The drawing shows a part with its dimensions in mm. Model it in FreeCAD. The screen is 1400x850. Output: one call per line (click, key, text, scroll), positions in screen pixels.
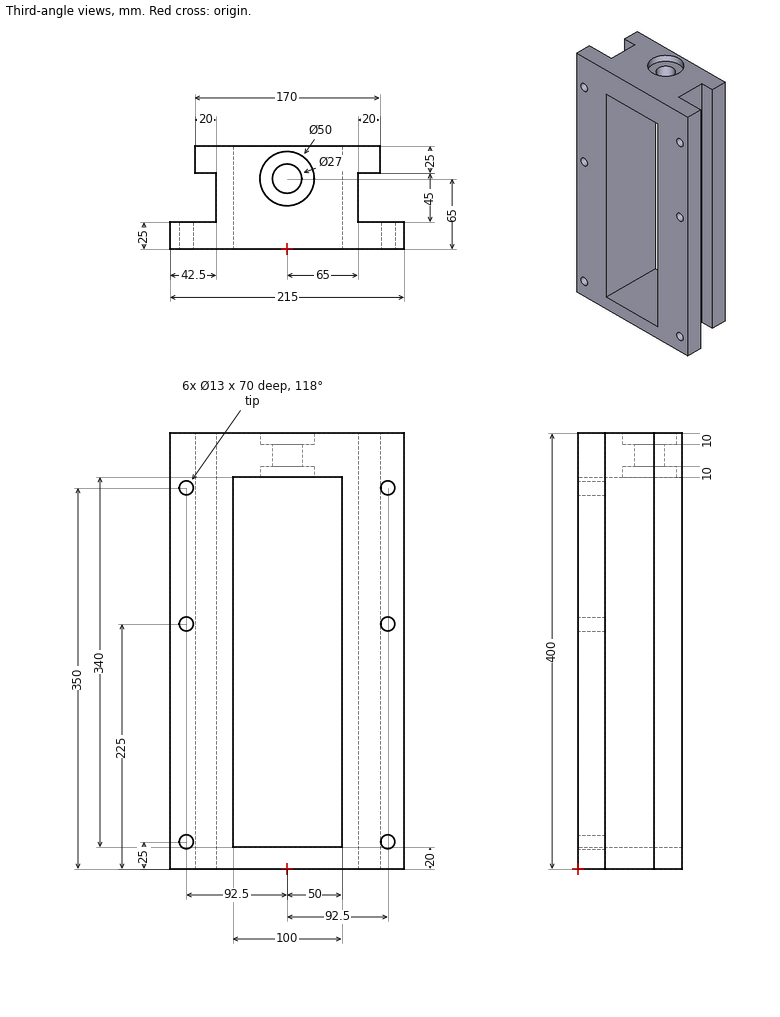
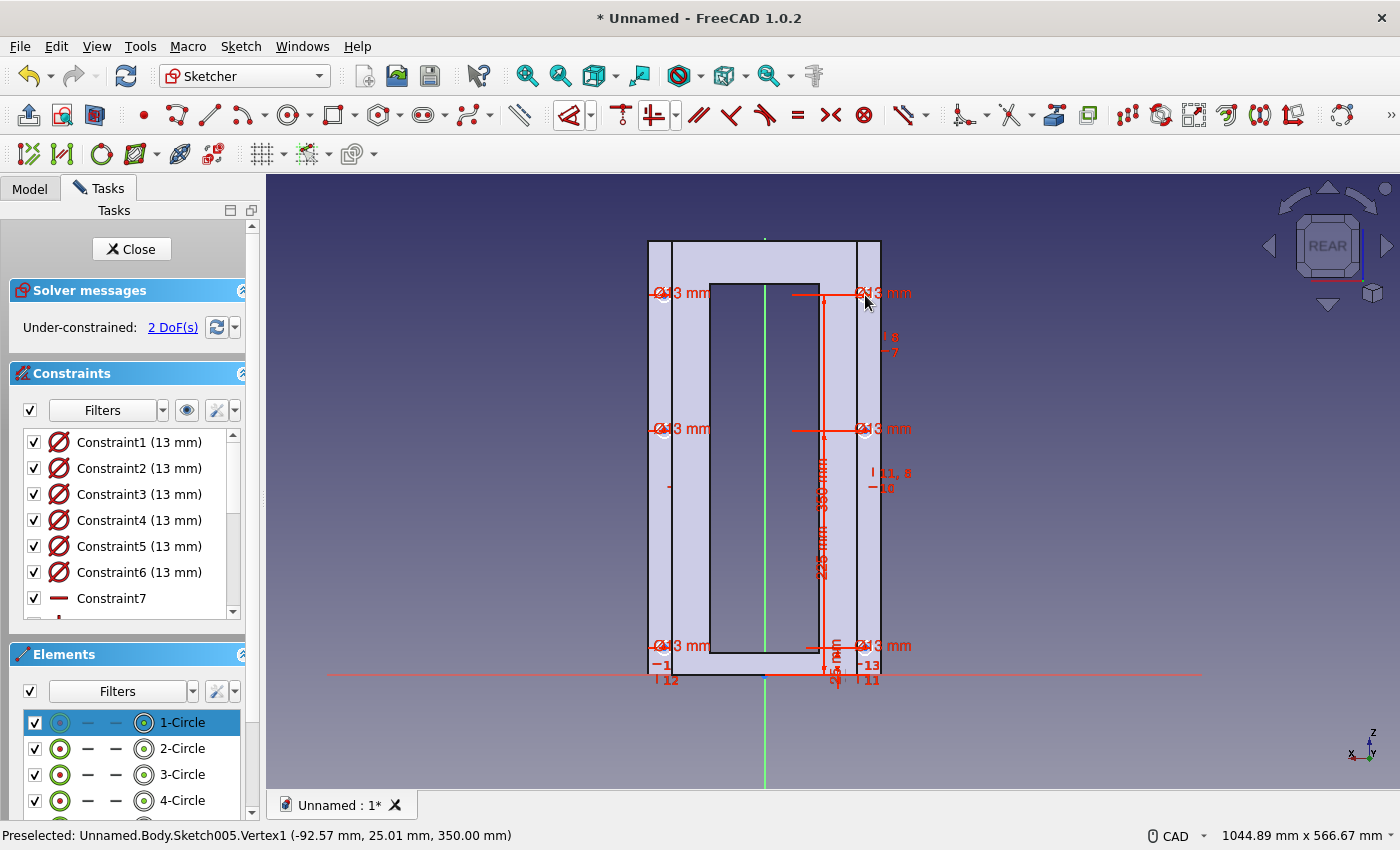
key(l)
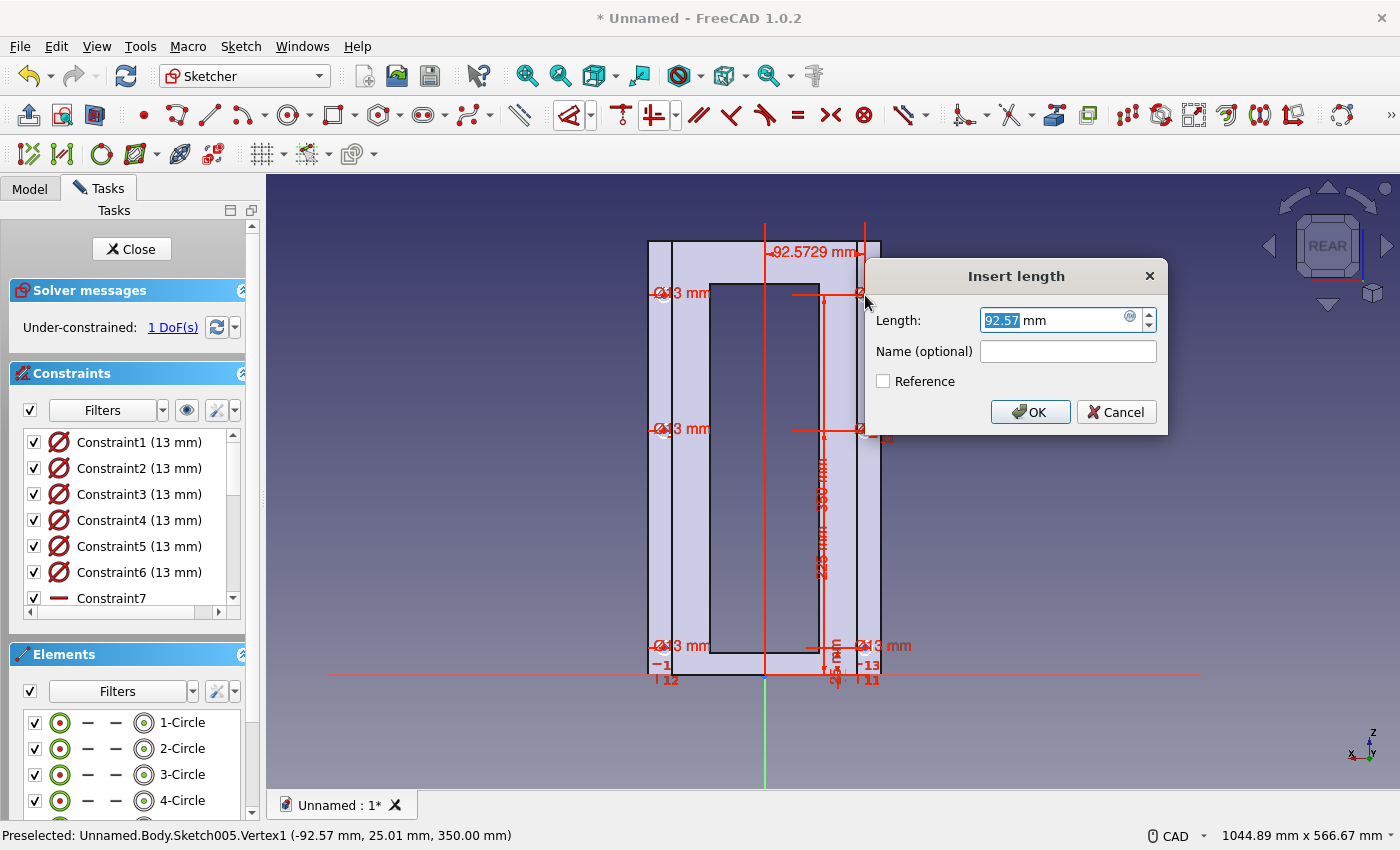
text(92.5)
key(Return)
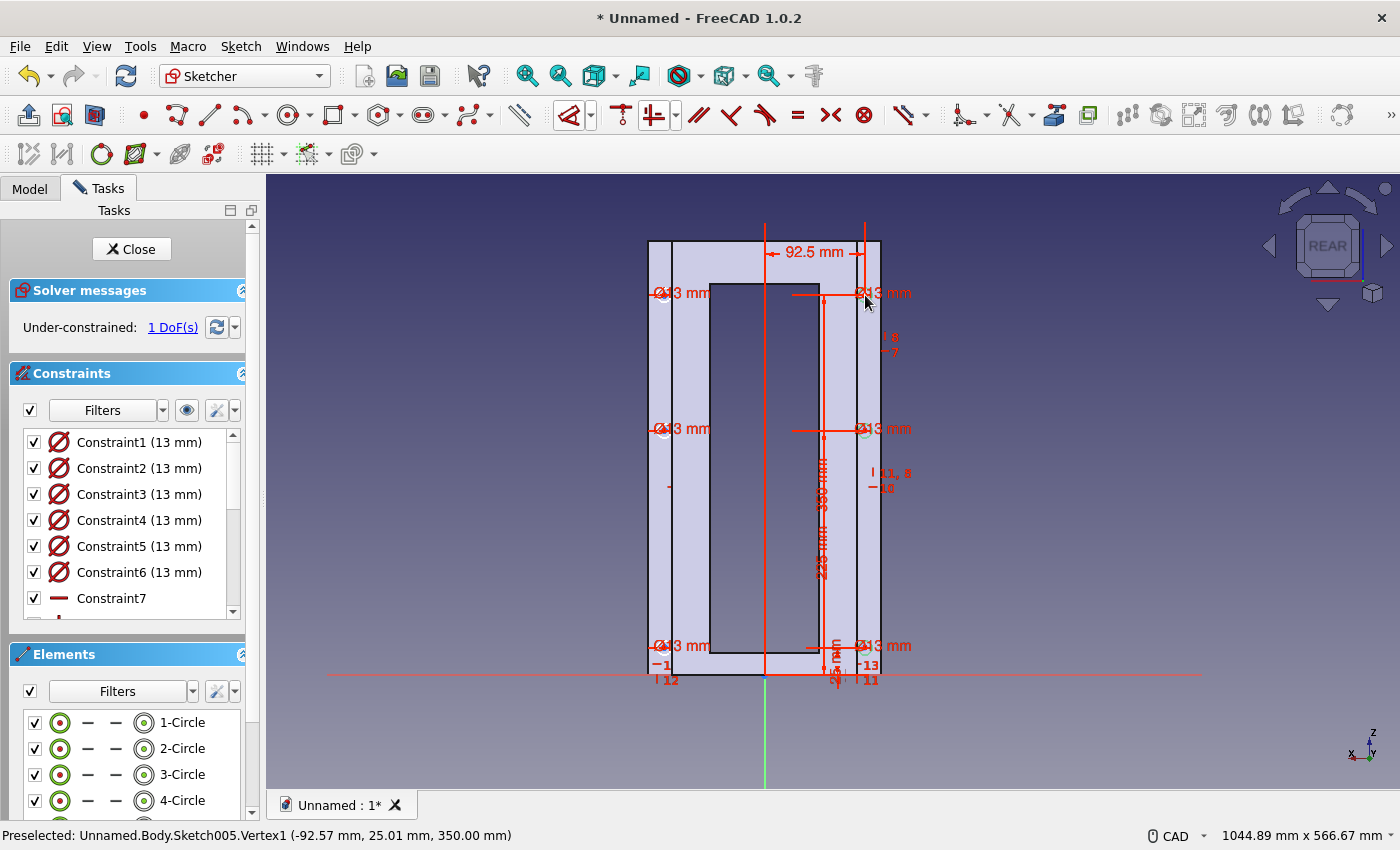
click(664, 295)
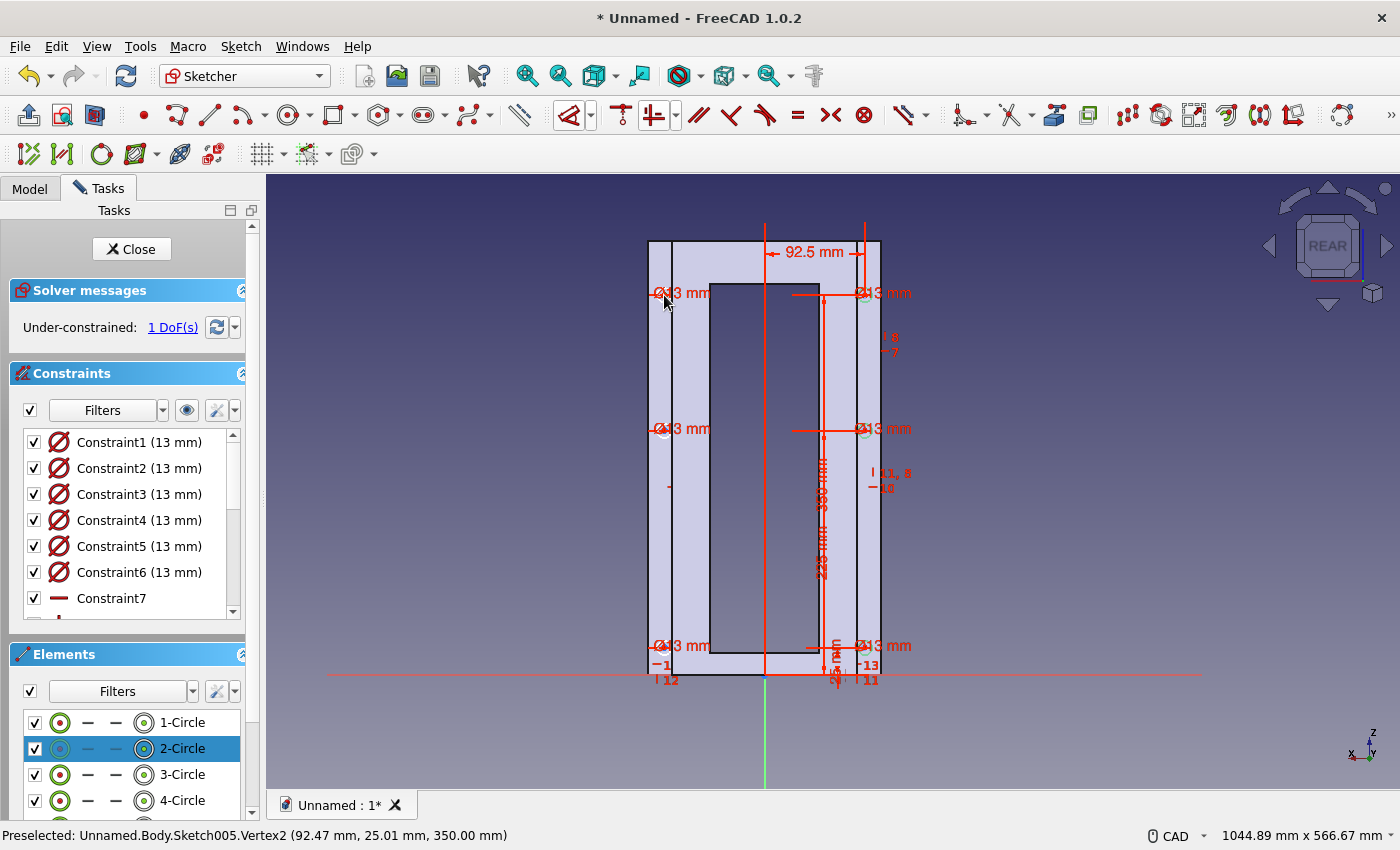
key(l)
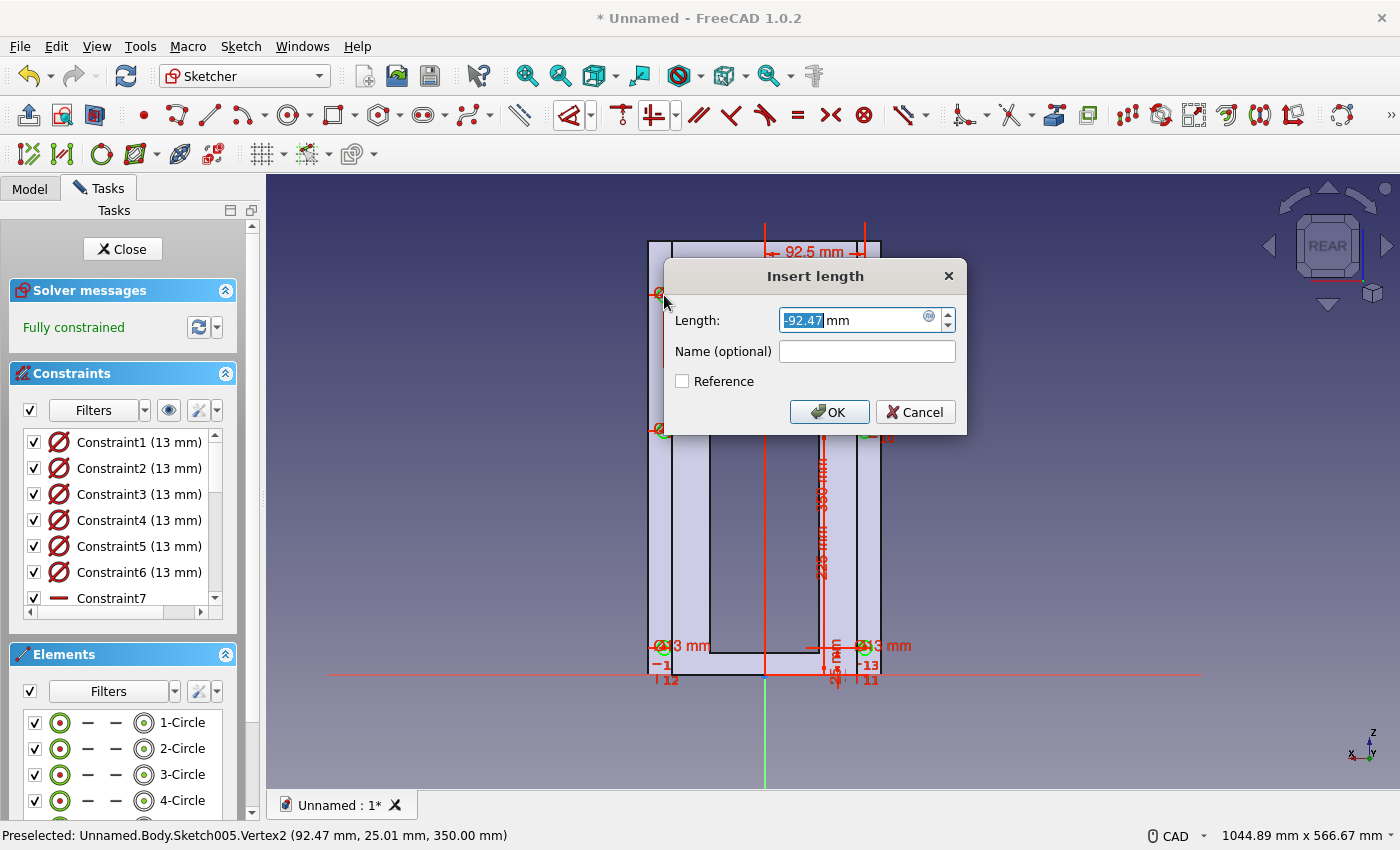
text(-92.5)
key(Return)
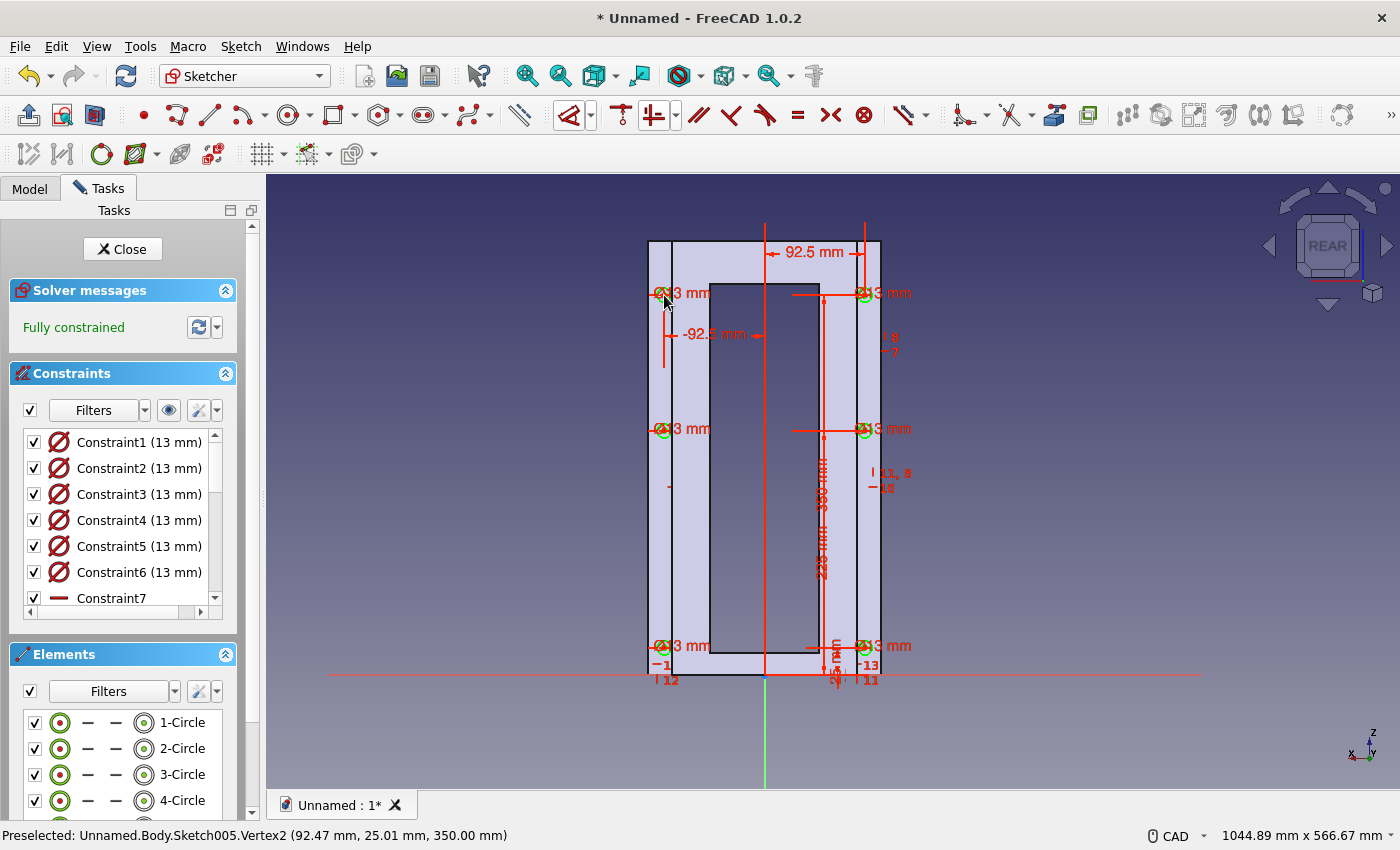
click(123, 249)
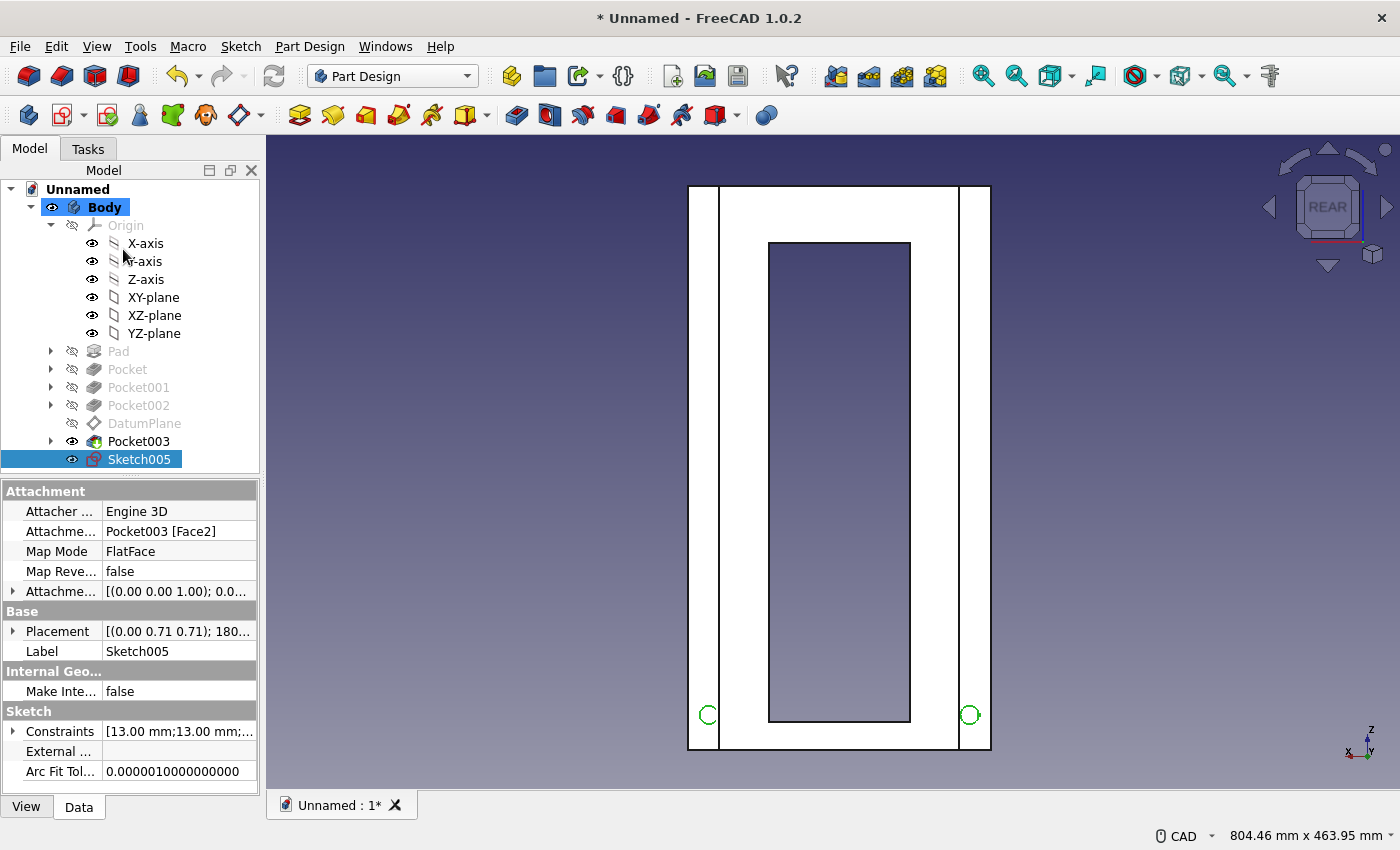
click(550, 116)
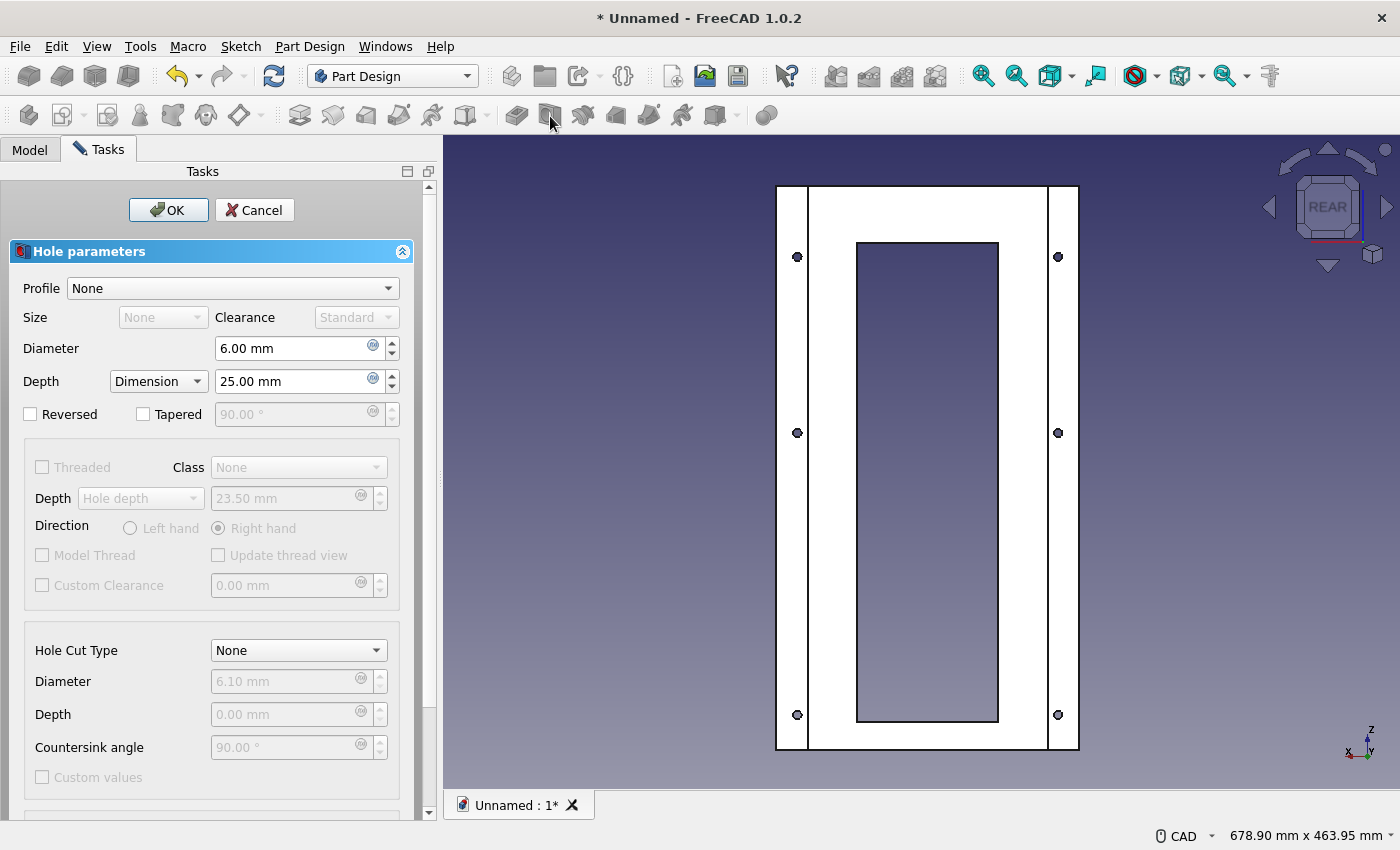
triple_click(300, 348)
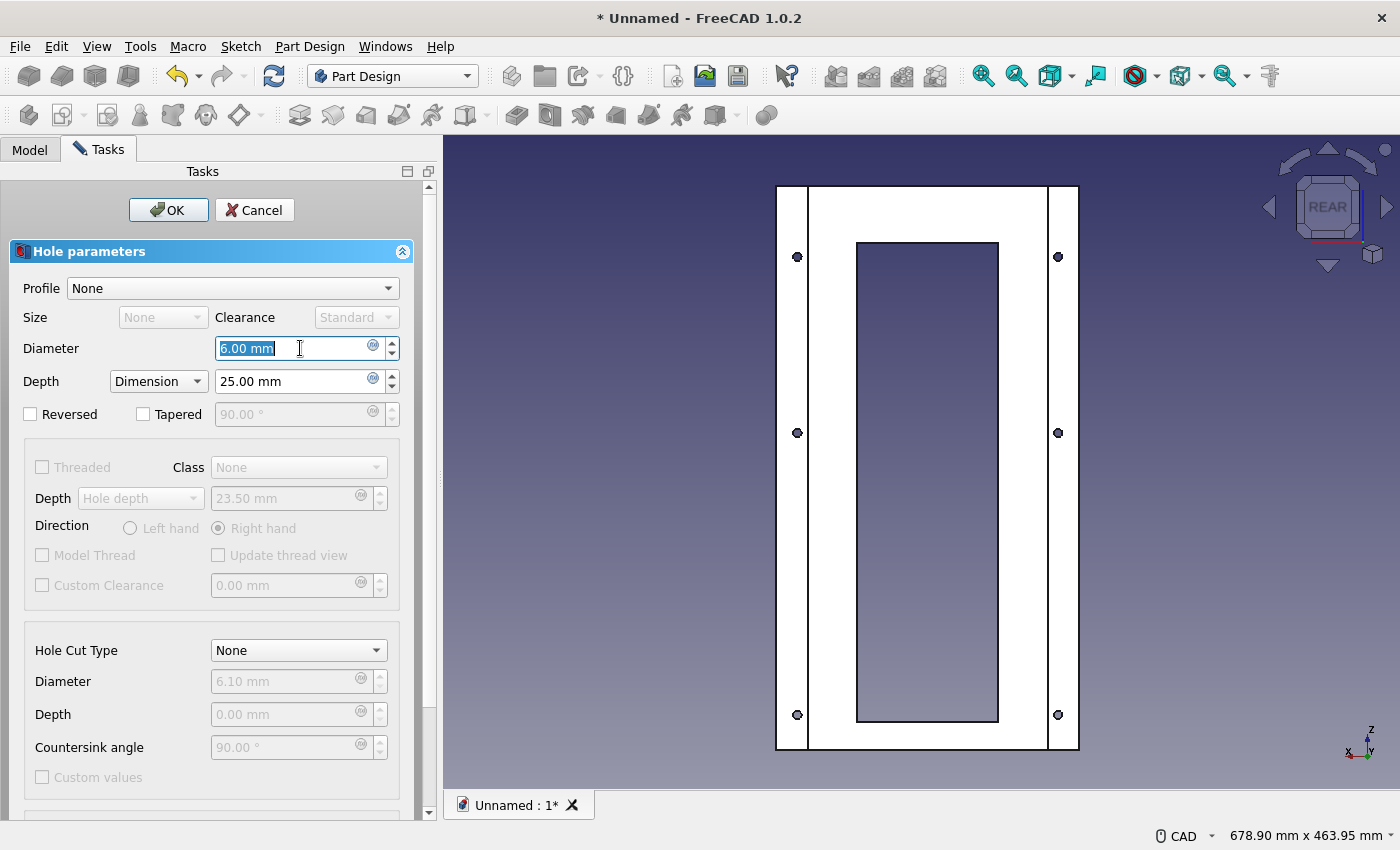
text(13)
key(Tab)